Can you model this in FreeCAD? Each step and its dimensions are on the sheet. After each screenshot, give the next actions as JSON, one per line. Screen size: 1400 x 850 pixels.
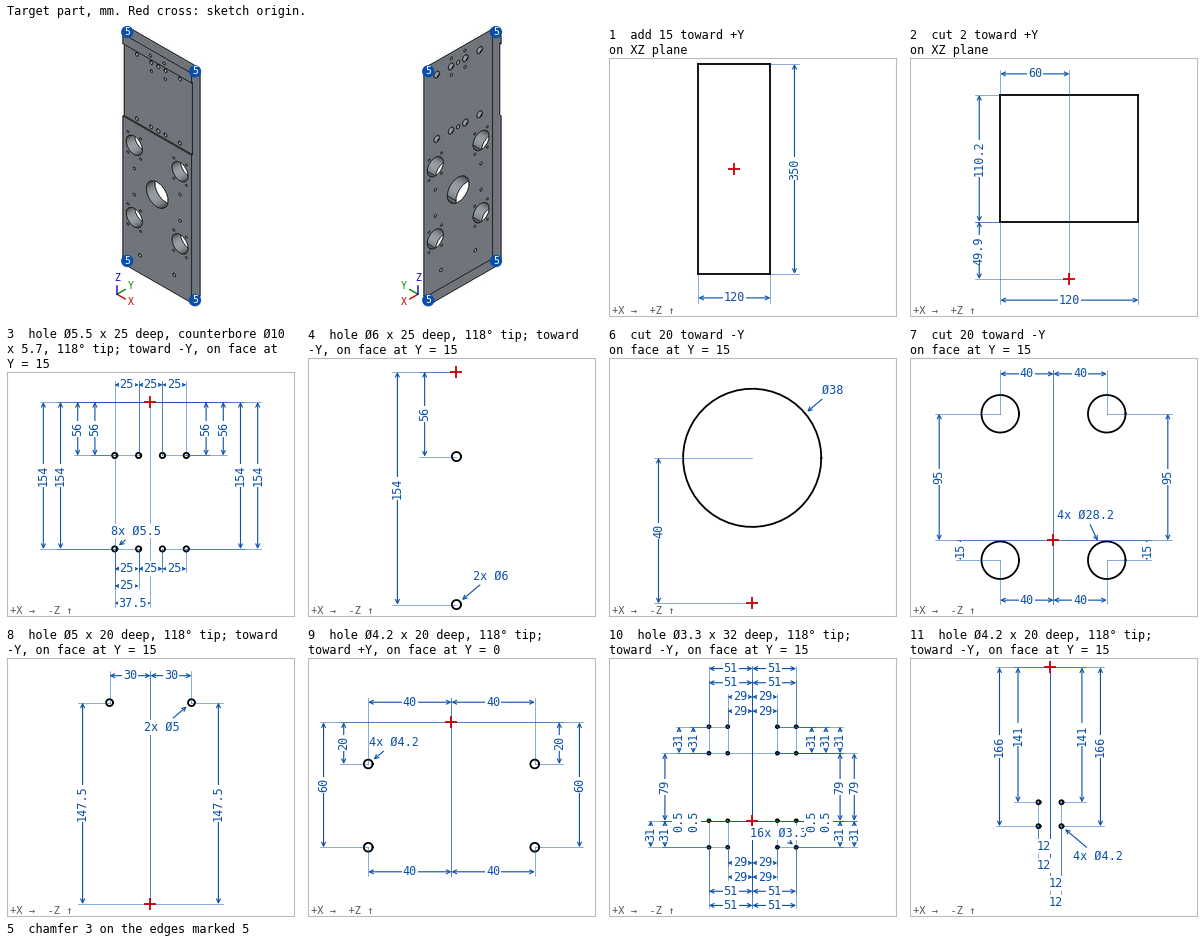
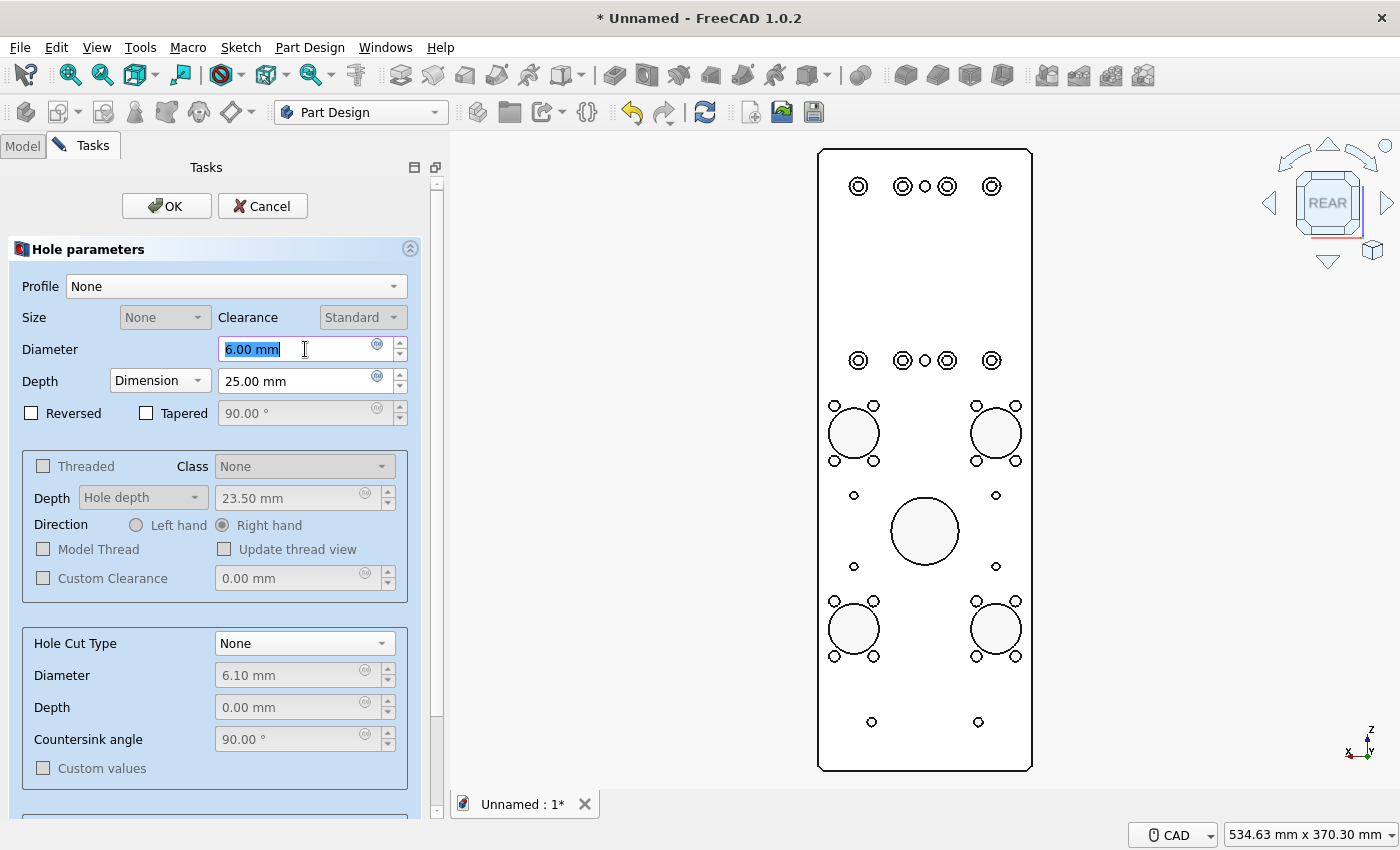
{"action": "type", "text": "3.3"}
{"action": "key", "text": "Tab"}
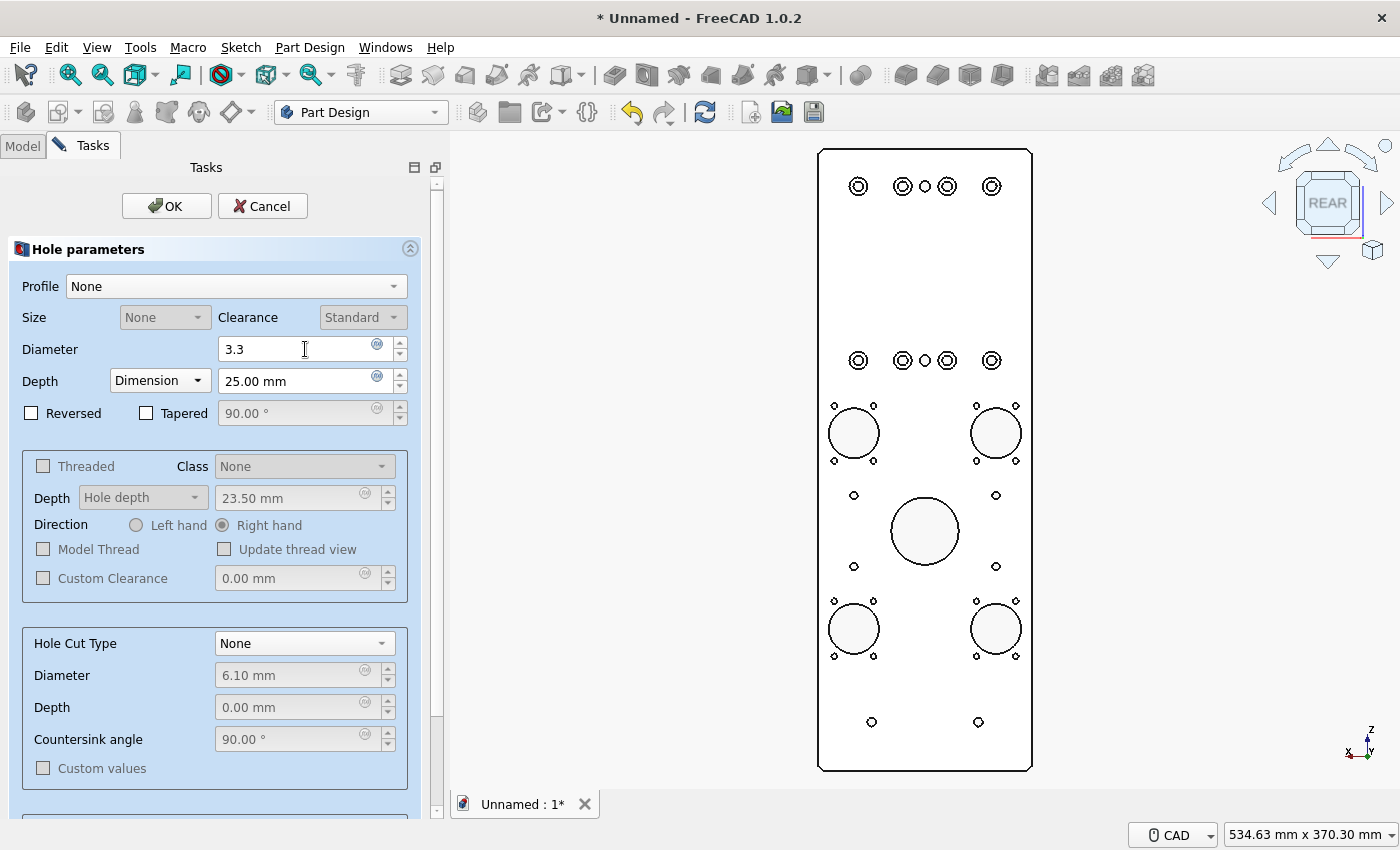
{"action": "triple_click", "coordinate": [305, 381]}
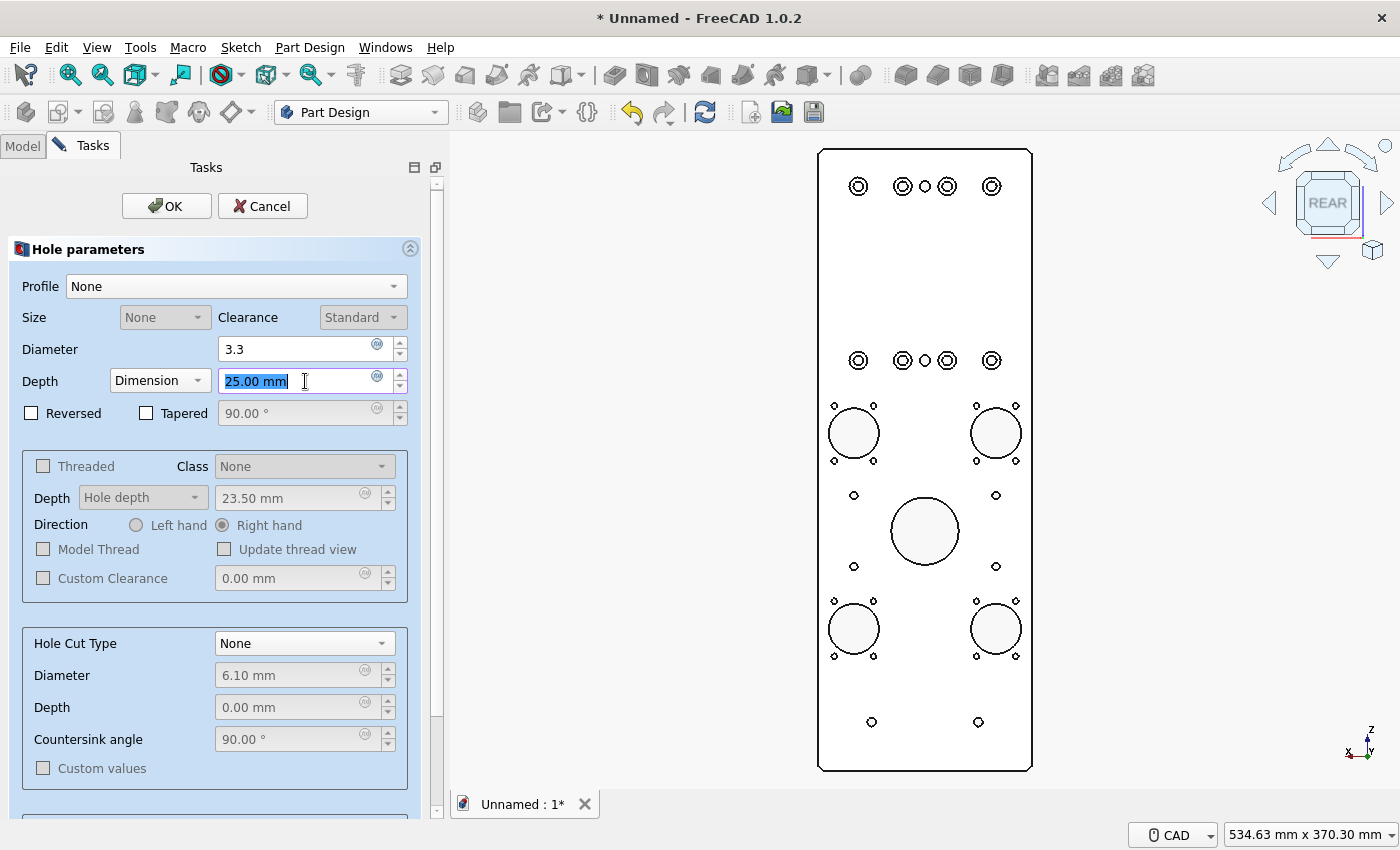
{"action": "type", "text": "32"}
{"action": "key", "text": "Tab"}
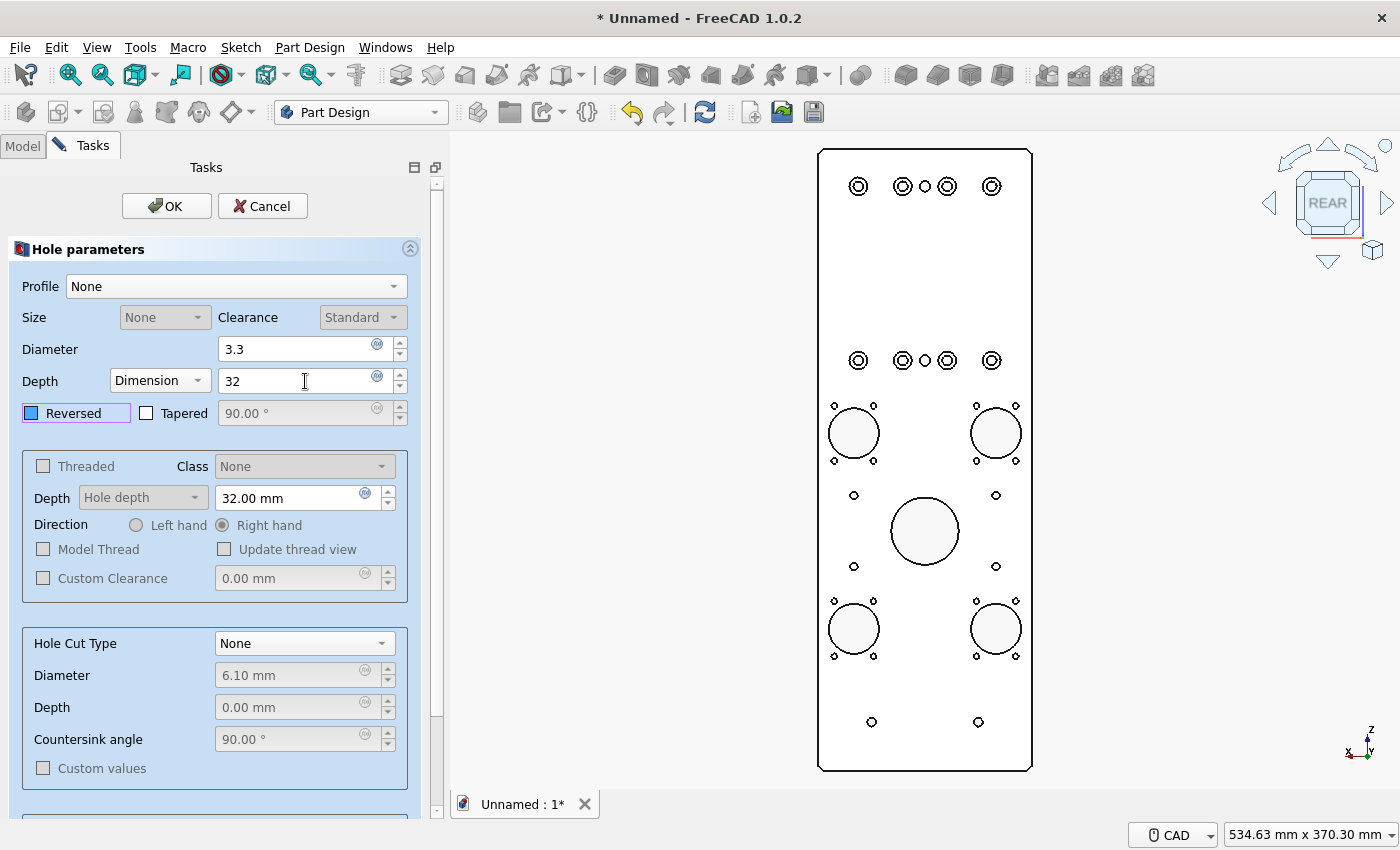
{"action": "left_click", "coordinate": [167, 206]}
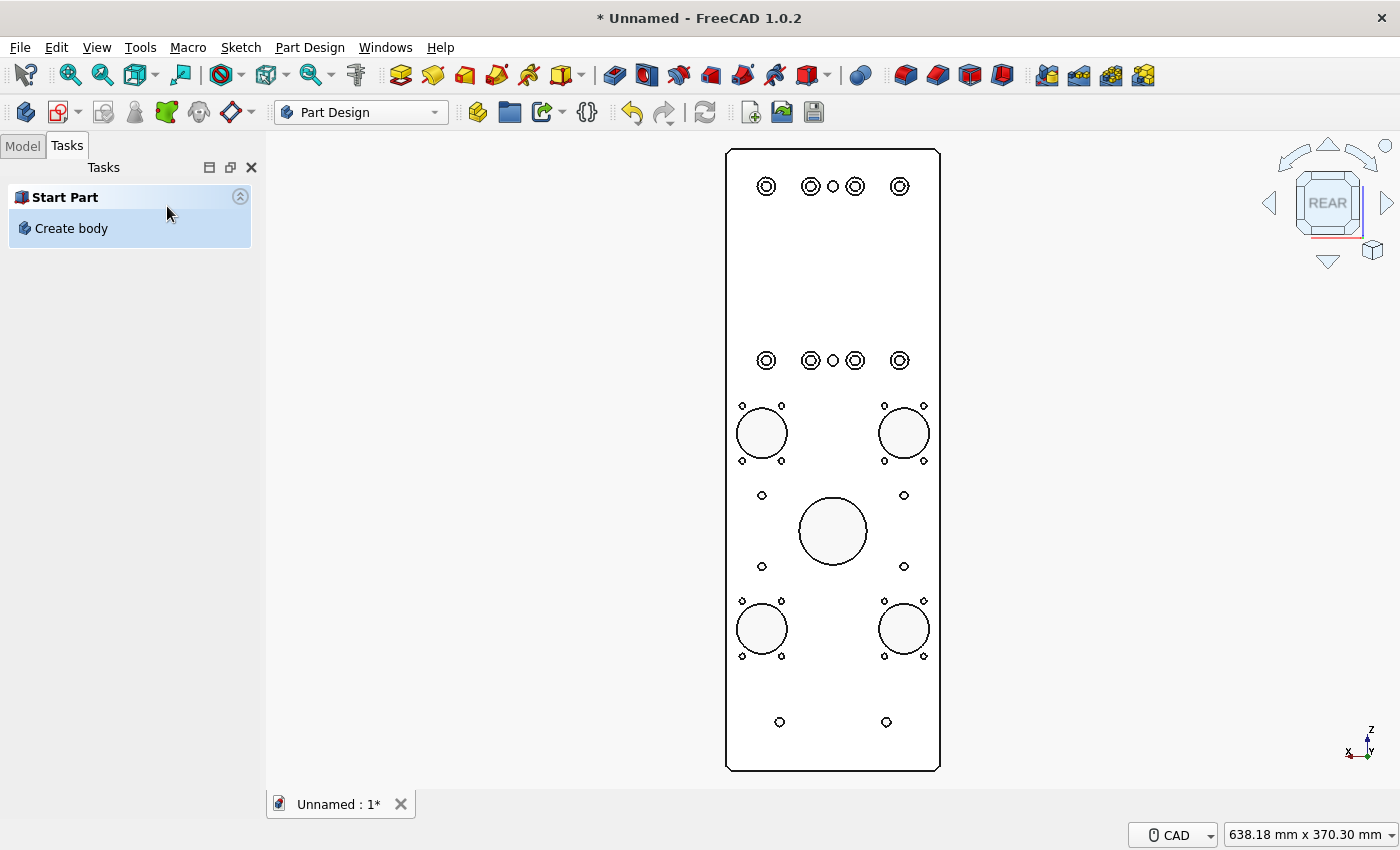
{"action": "left_click", "coordinate": [833, 281]}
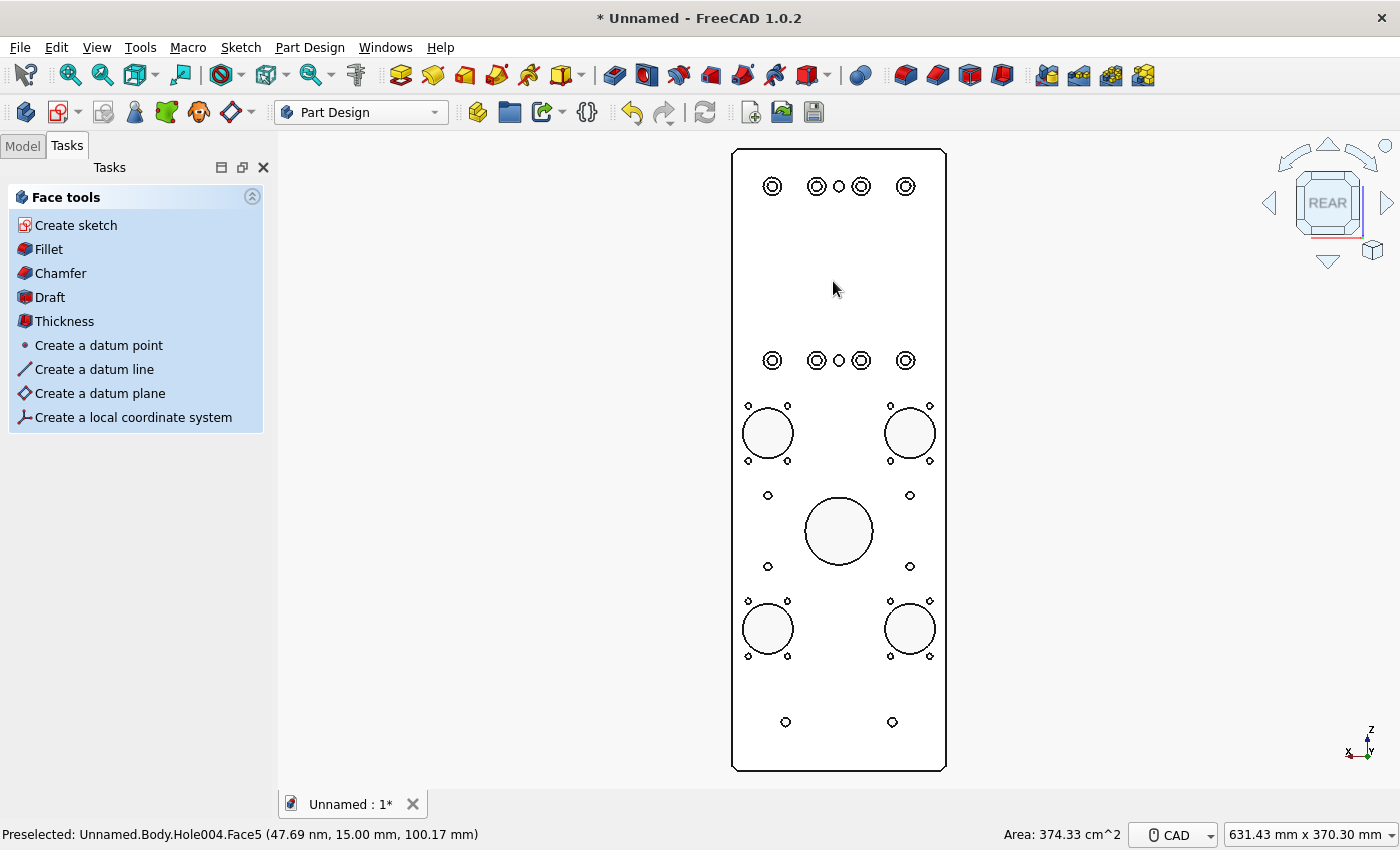
{"action": "left_click", "coordinate": [58, 112]}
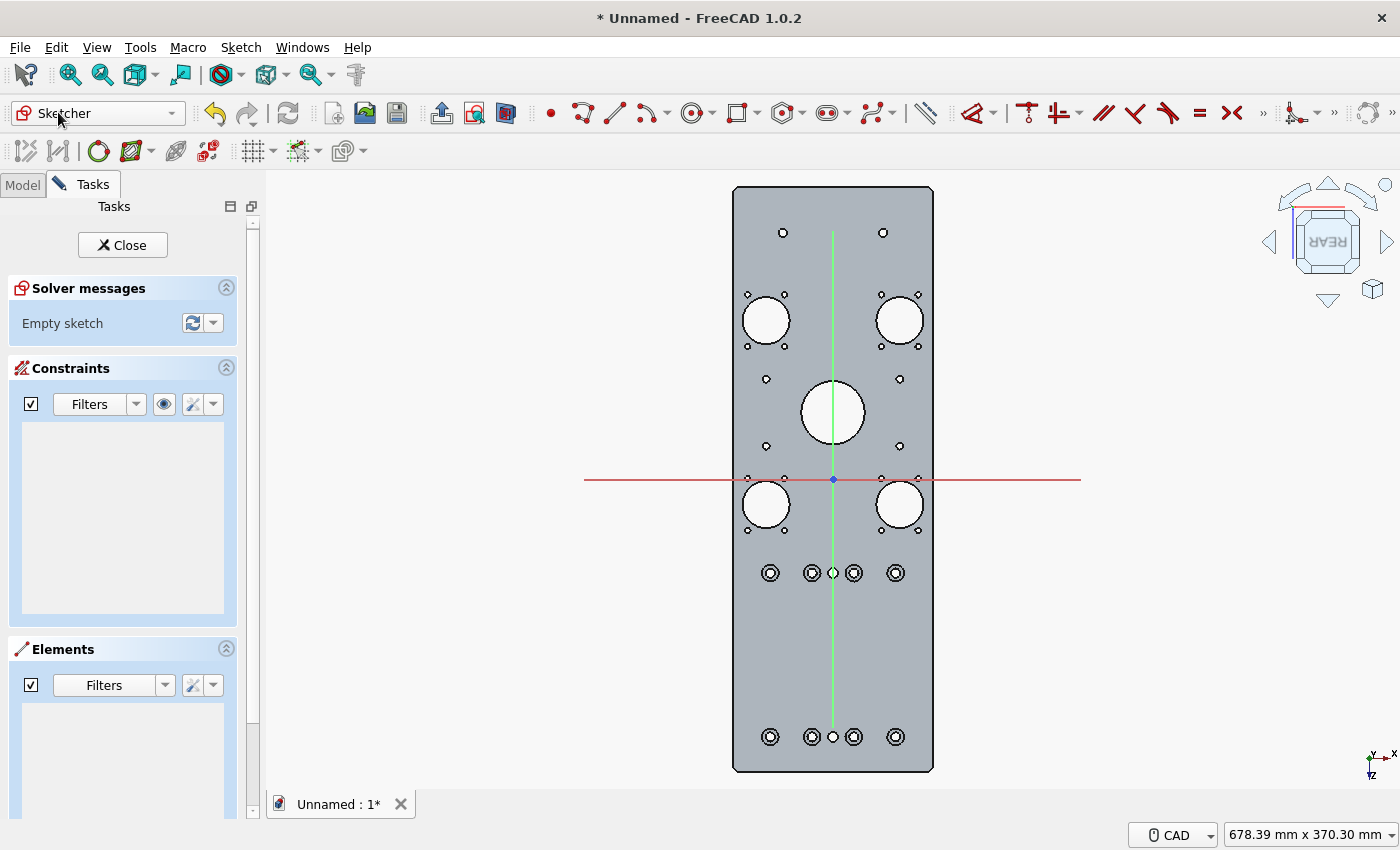
{"action": "scroll", "coordinate": [764, 480], "scroll_direction": "down", "scroll_amount": 5}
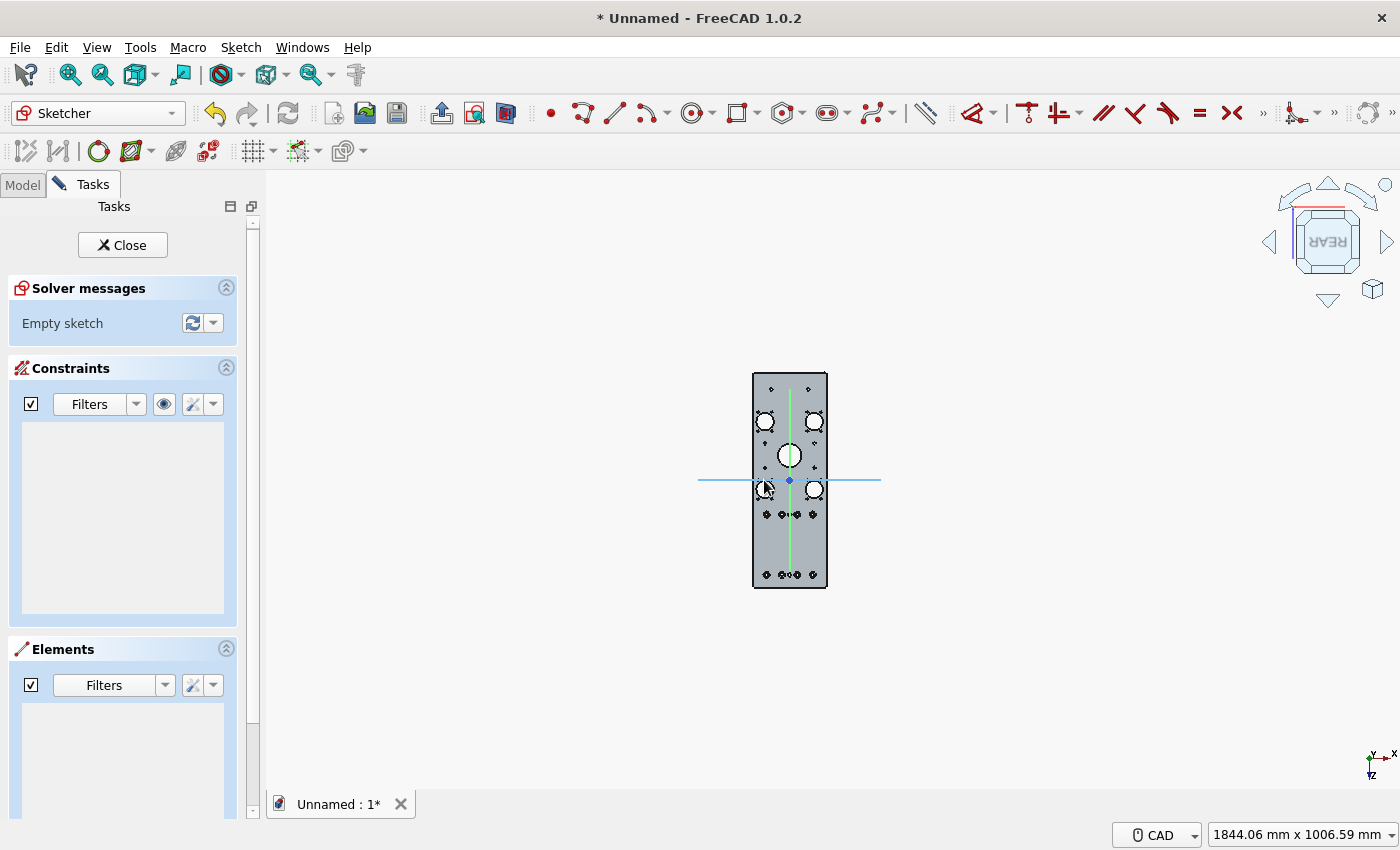
{"action": "scroll", "coordinate": [791, 580], "scroll_direction": "up", "scroll_amount": 15}